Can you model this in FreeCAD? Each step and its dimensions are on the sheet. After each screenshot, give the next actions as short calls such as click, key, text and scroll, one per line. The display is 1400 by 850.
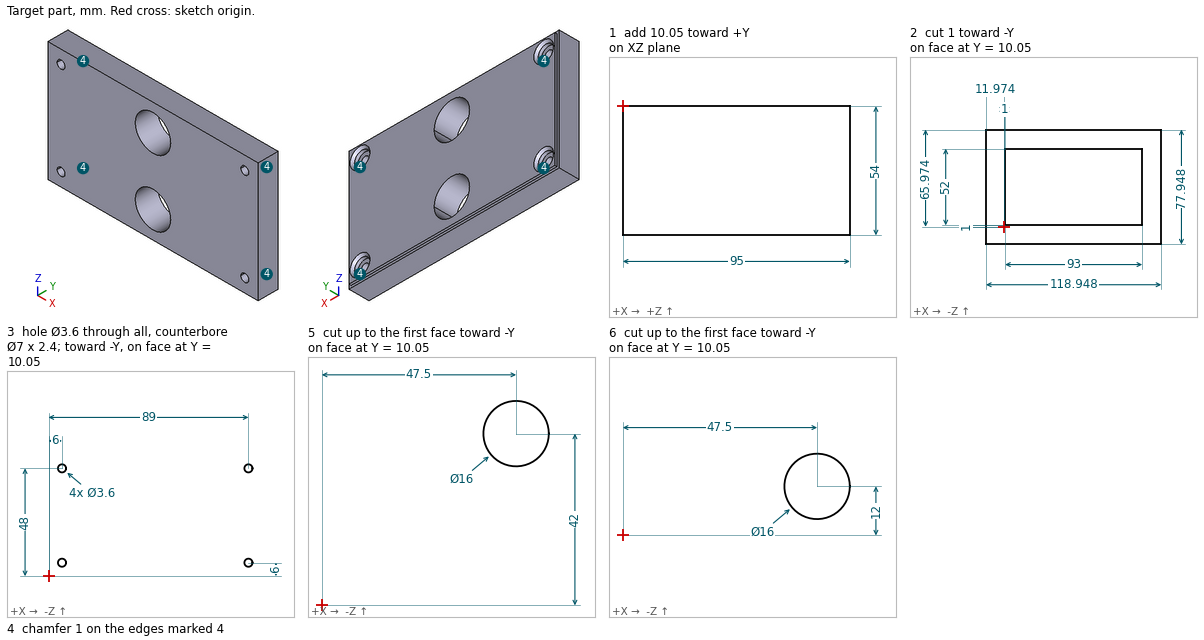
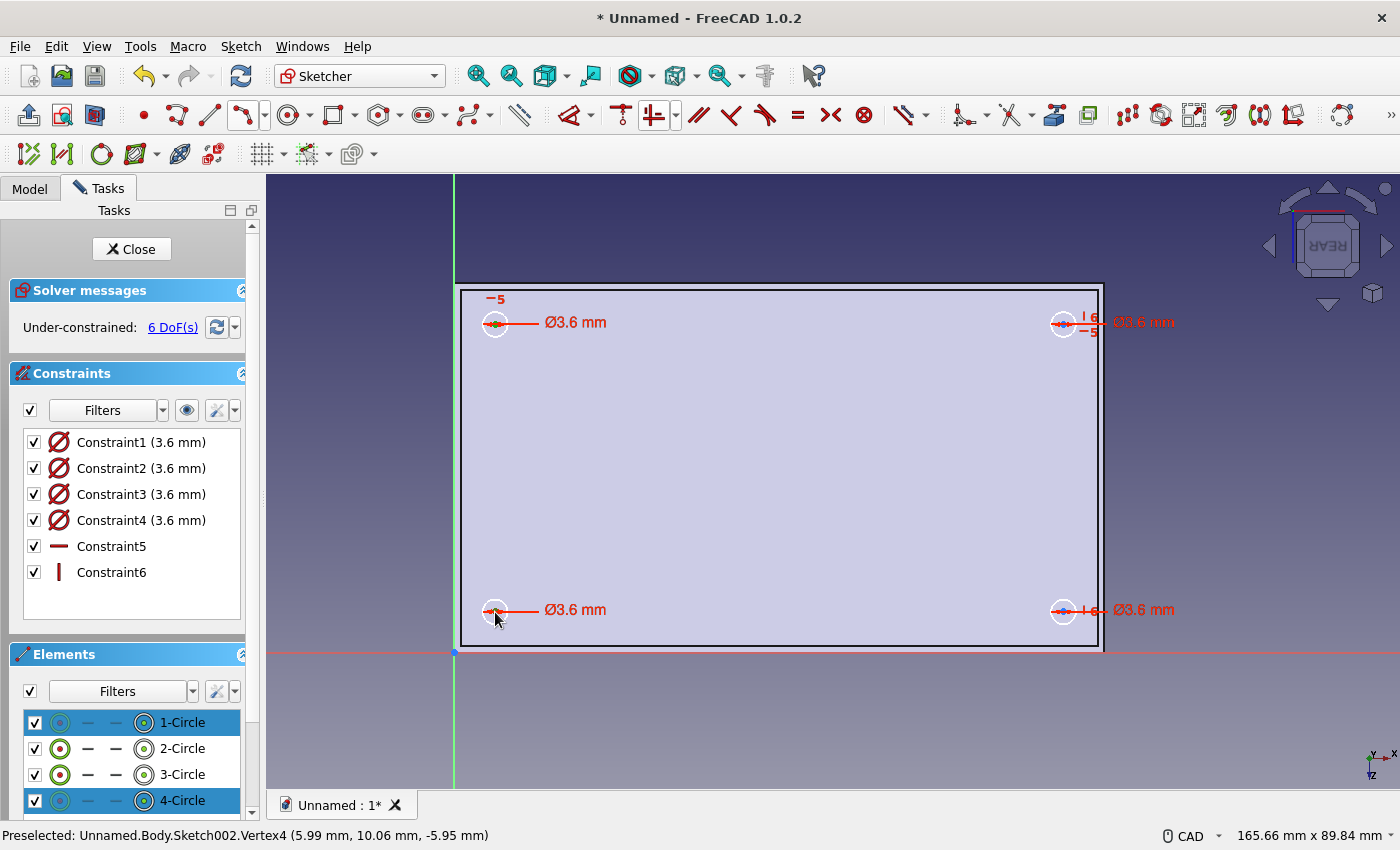
click(676, 116)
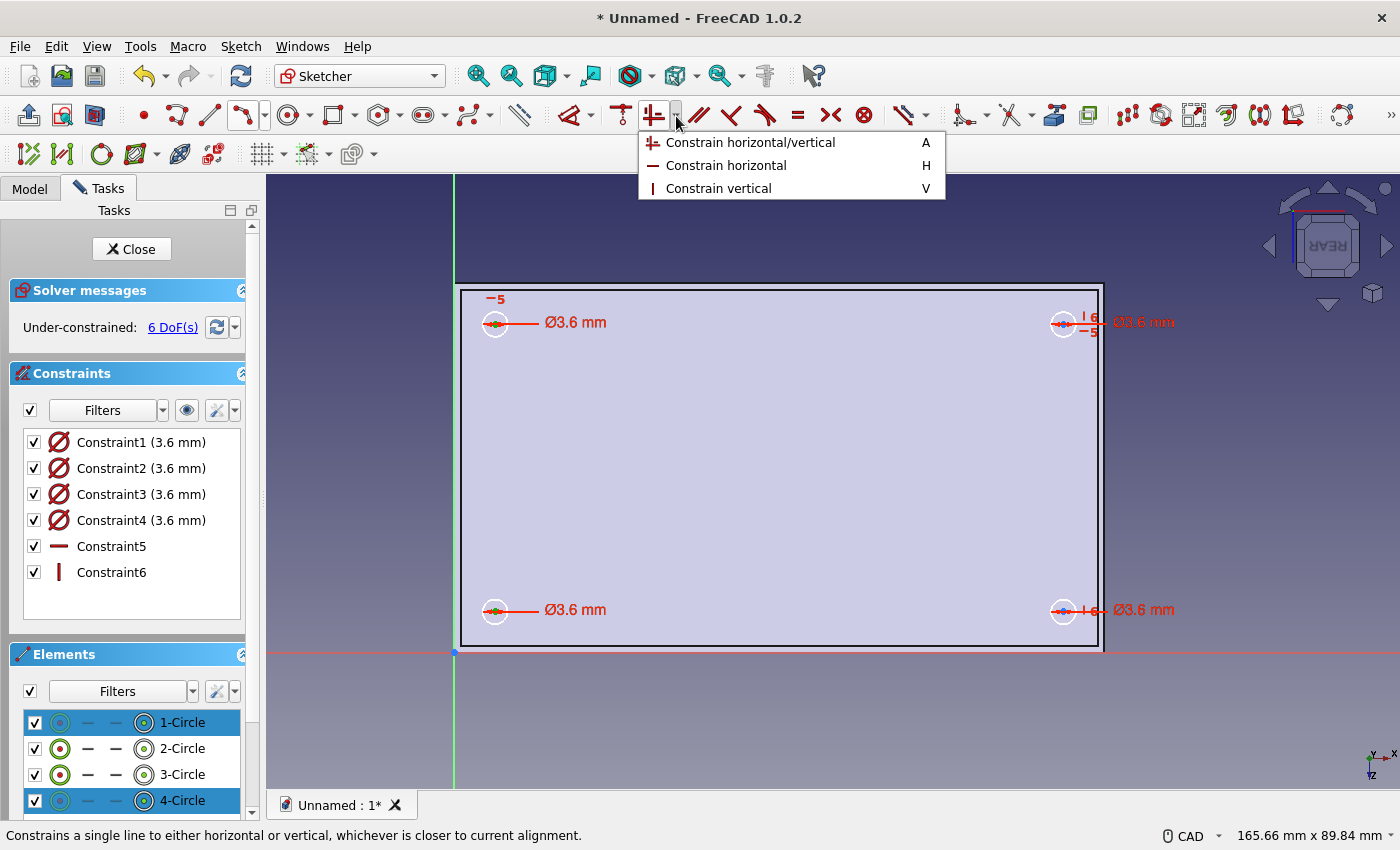
click(792, 188)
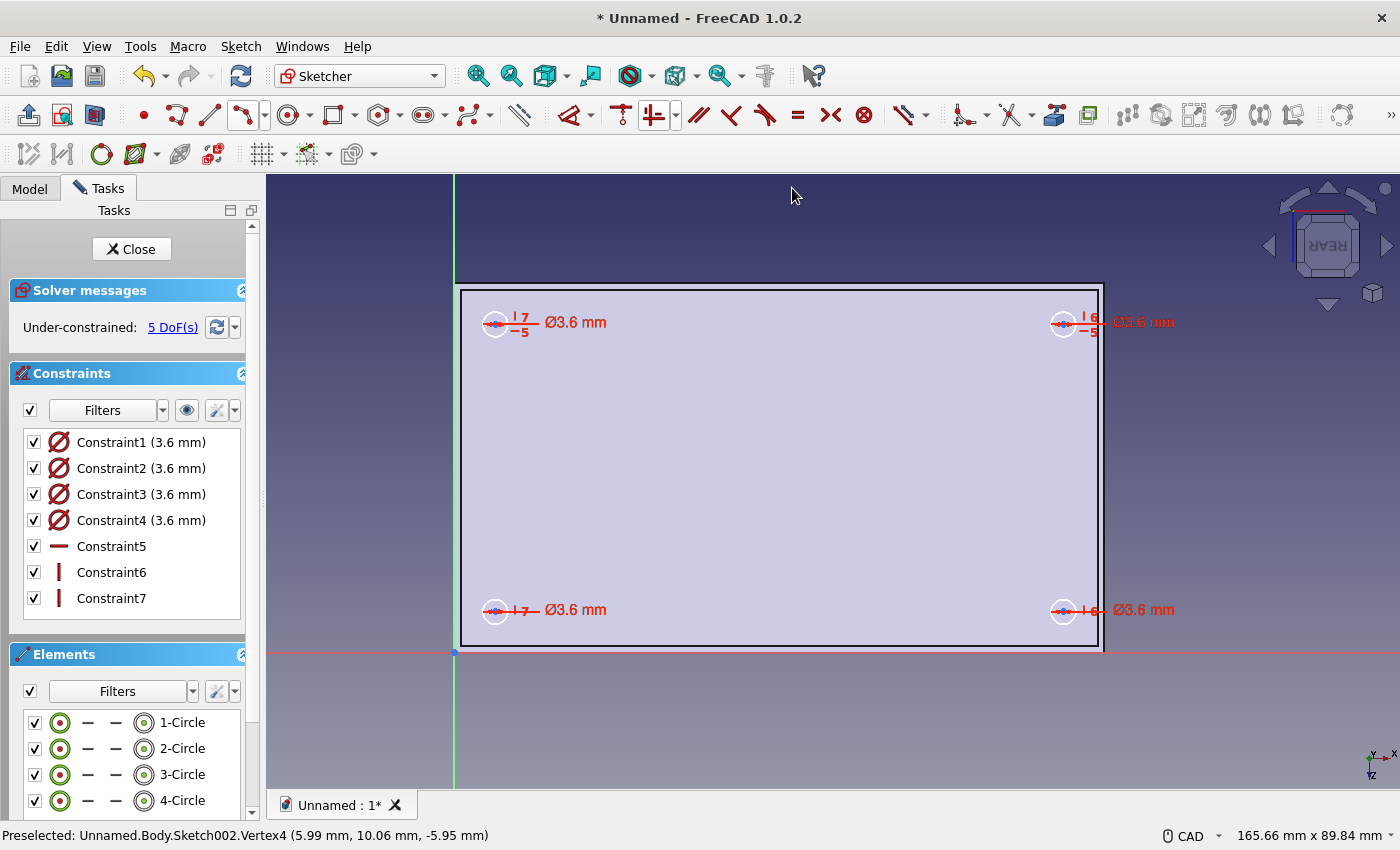
click(1063, 612)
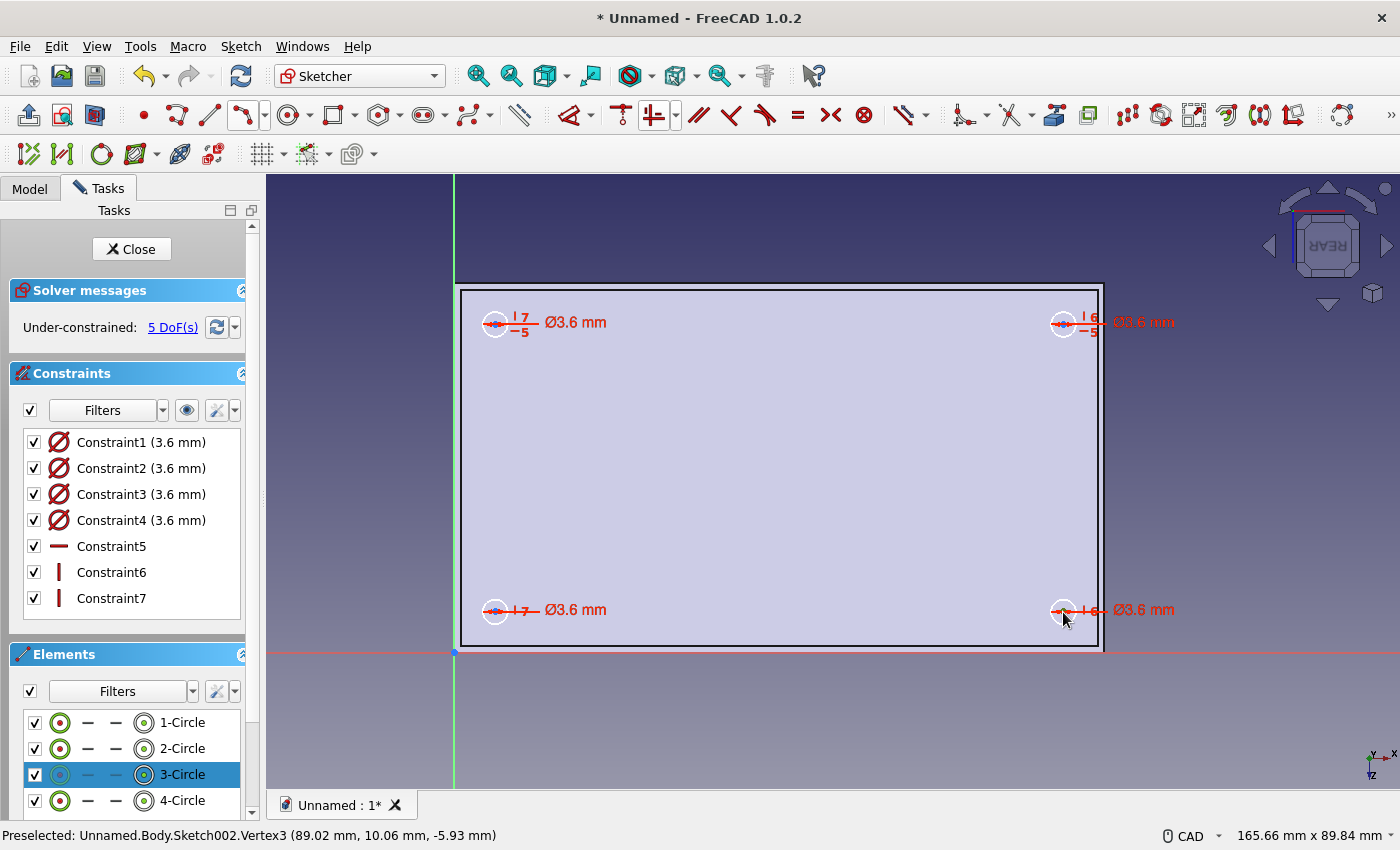
click(495, 612)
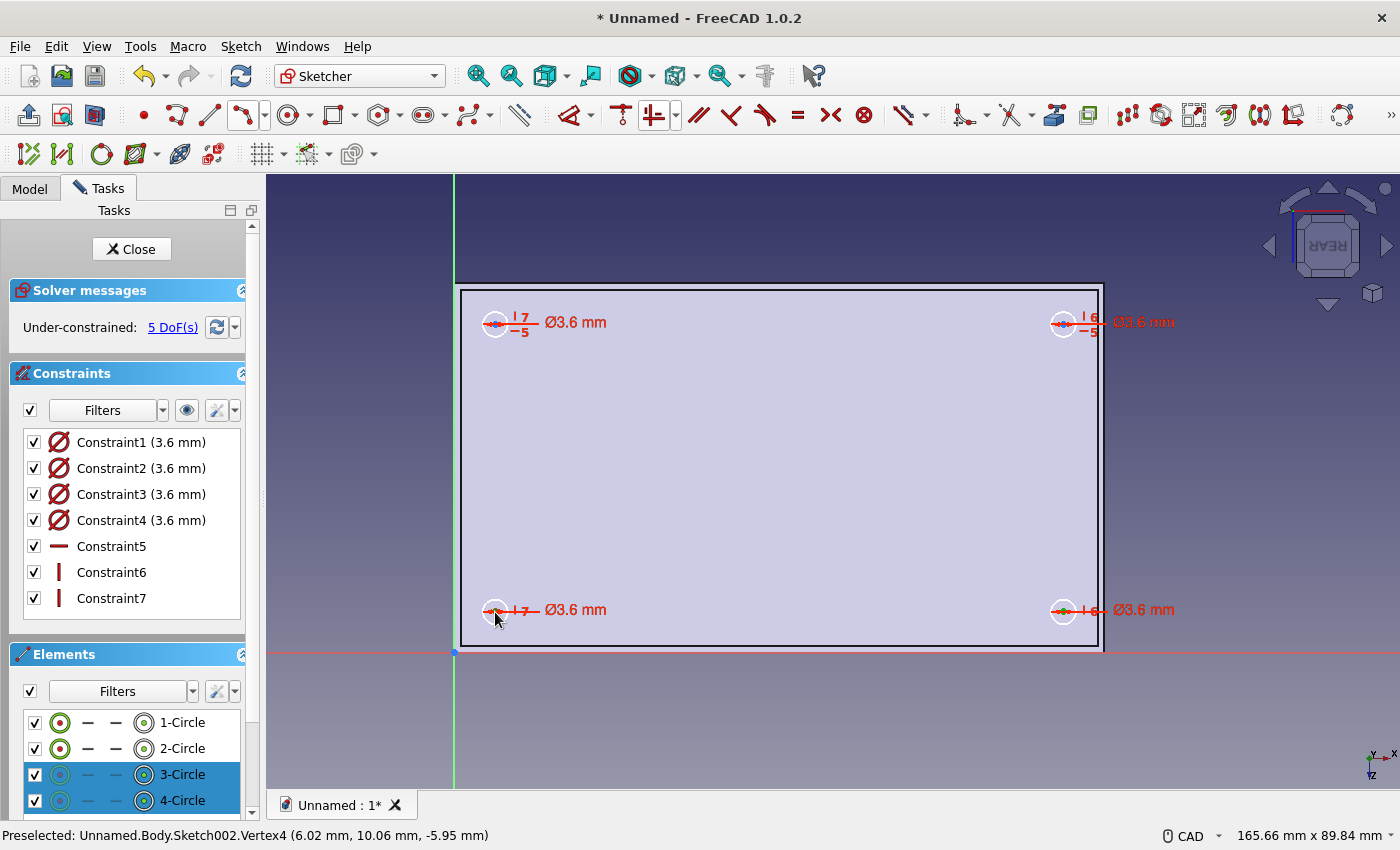
key(h)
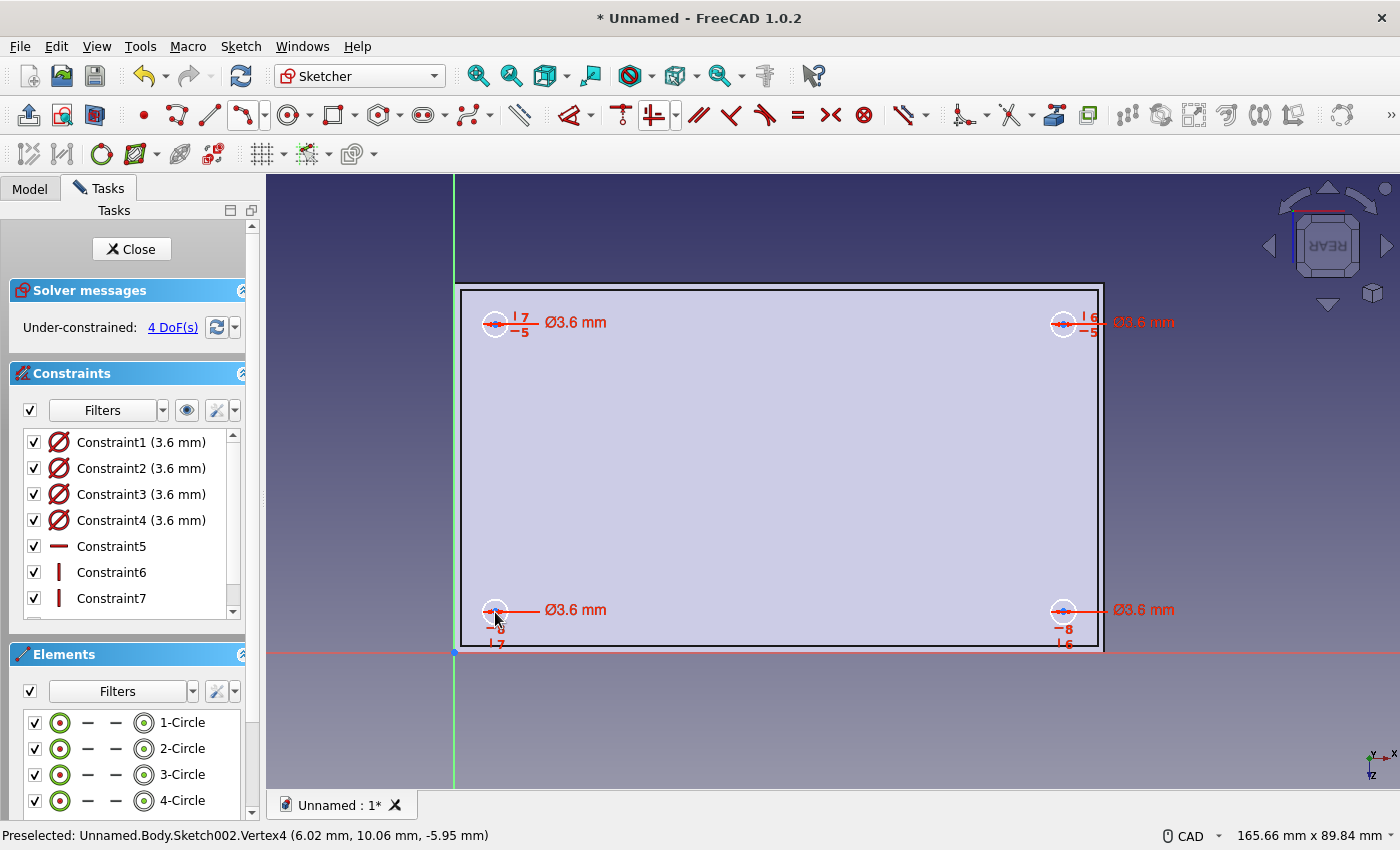
click(568, 116)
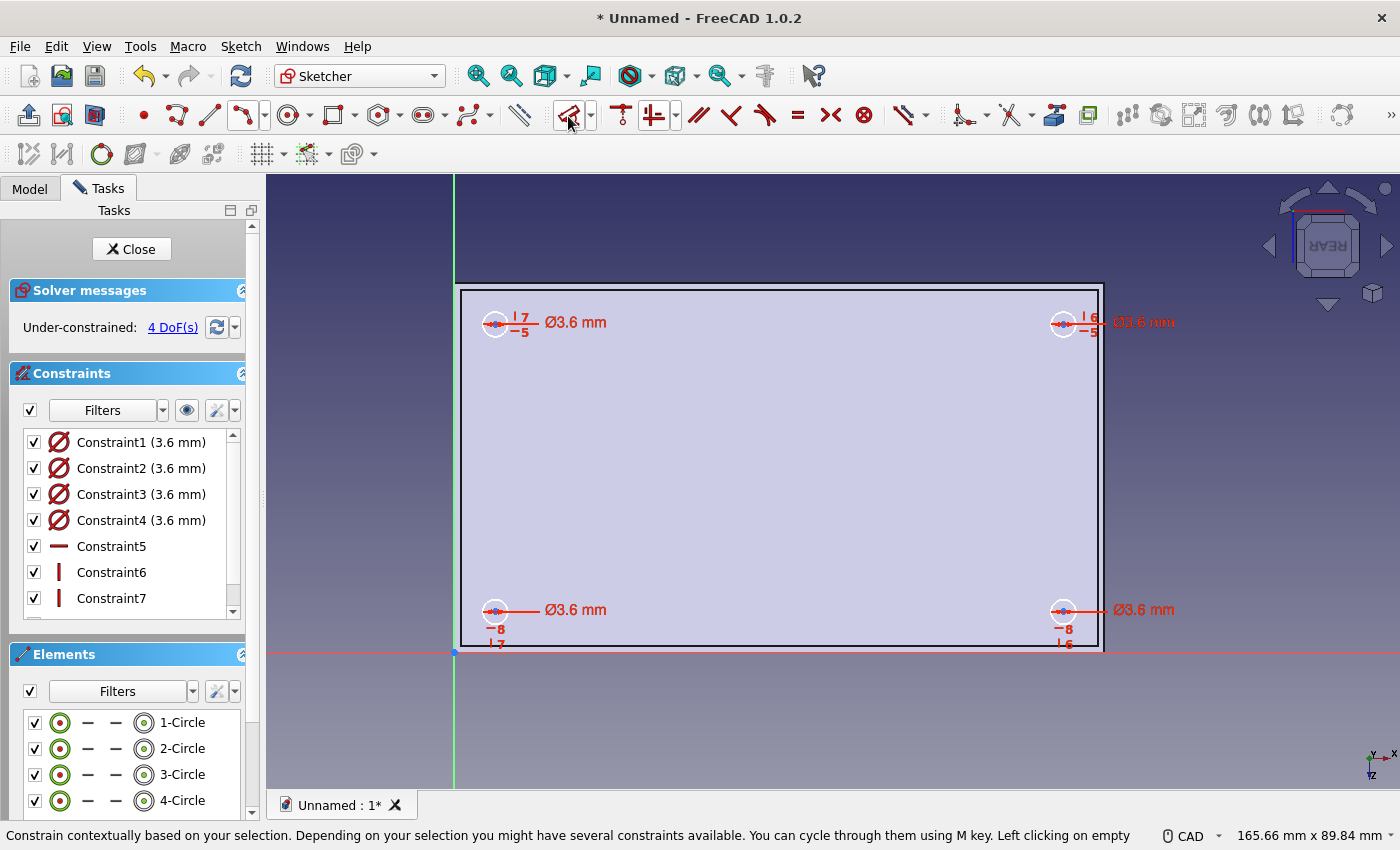
click(495, 324)
click(475, 687)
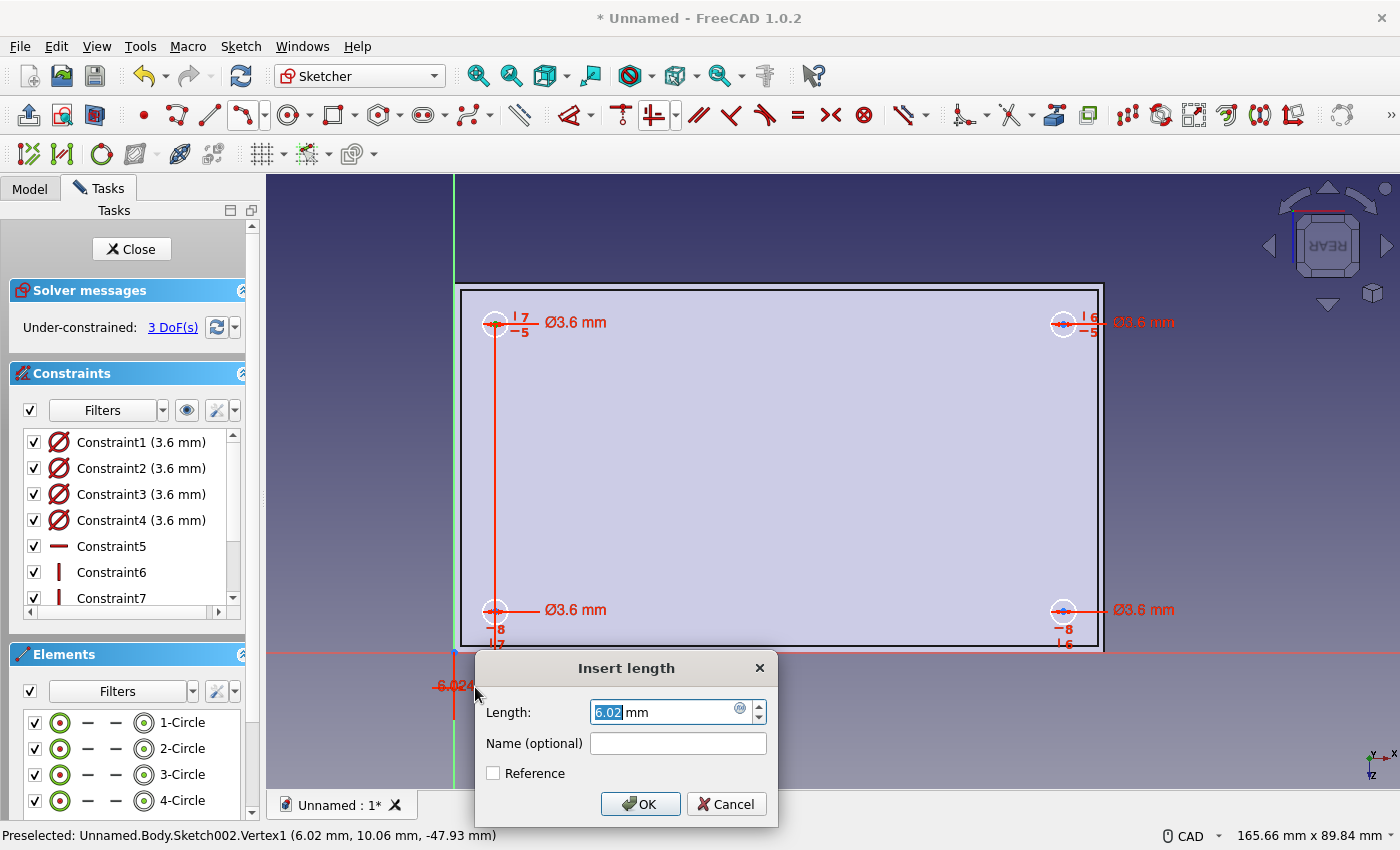
text(6)
key(Return)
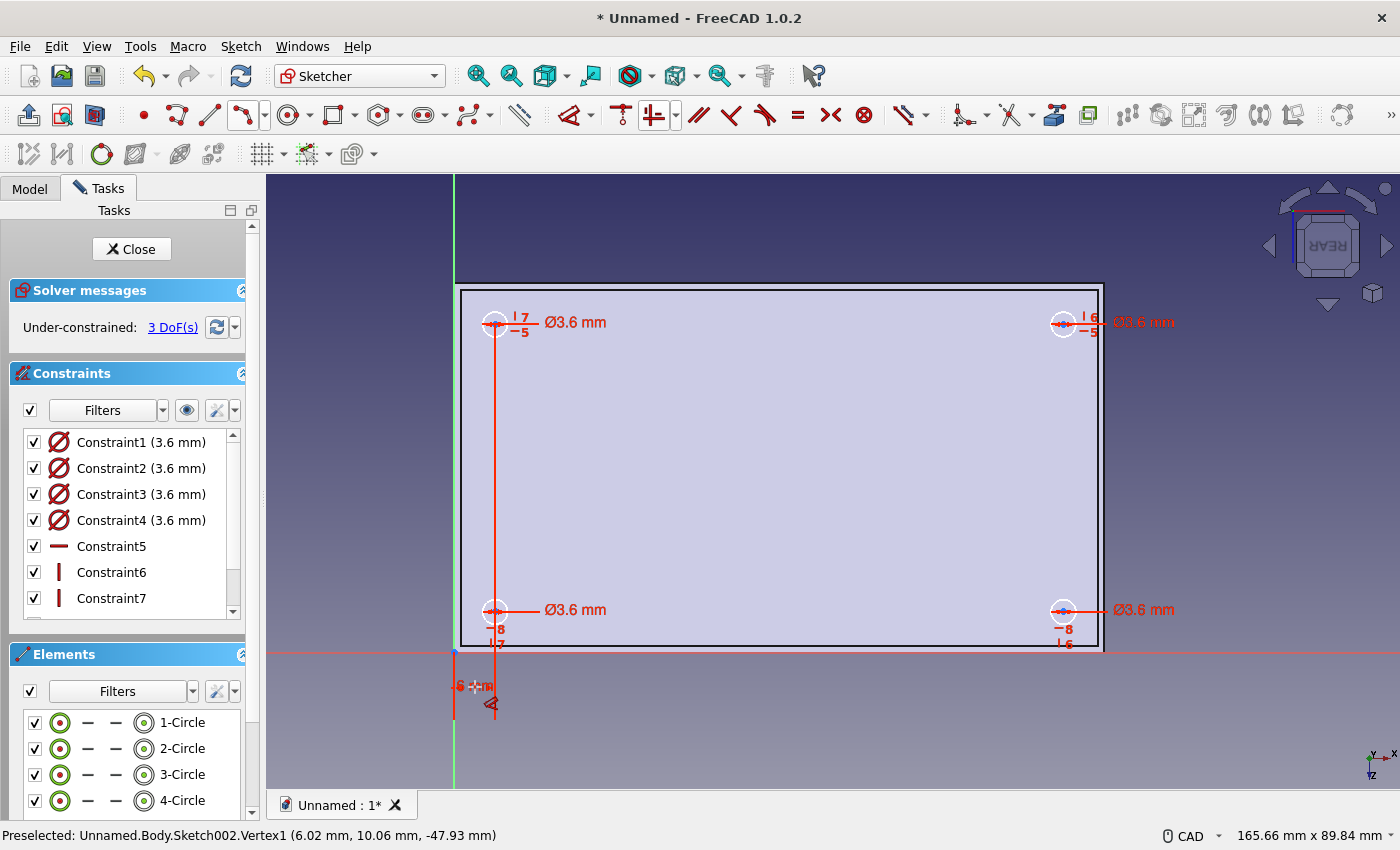
click(1063, 612)
click(420, 632)